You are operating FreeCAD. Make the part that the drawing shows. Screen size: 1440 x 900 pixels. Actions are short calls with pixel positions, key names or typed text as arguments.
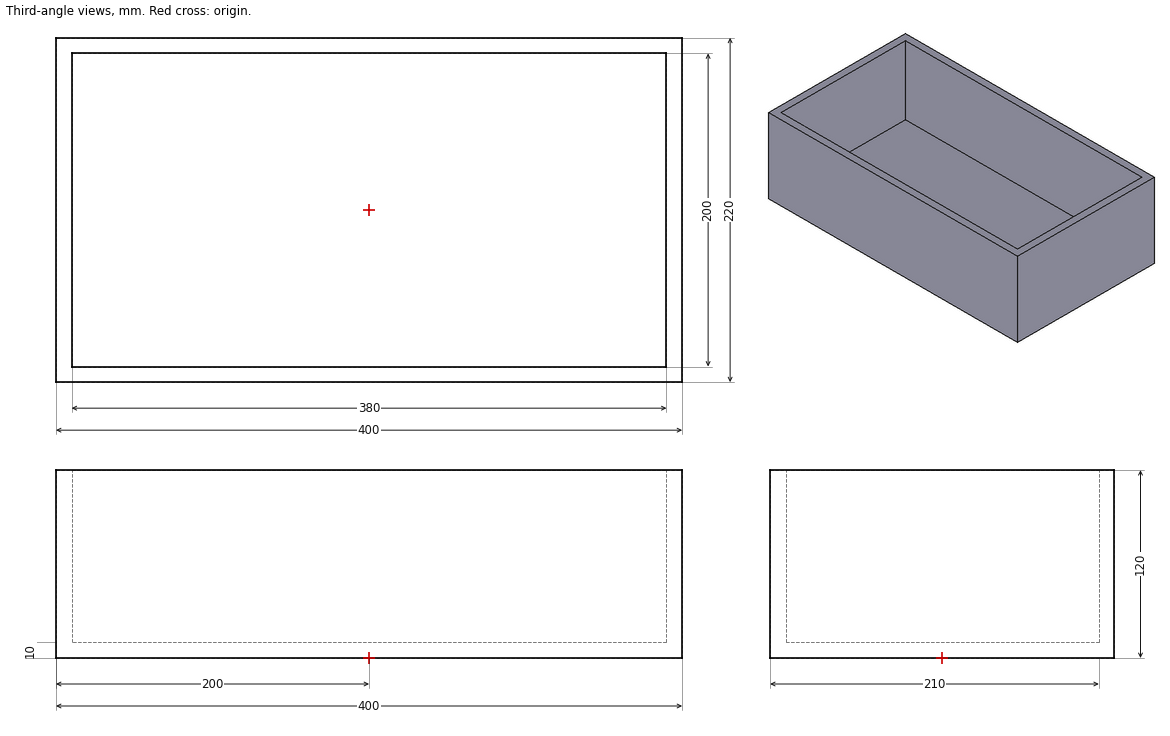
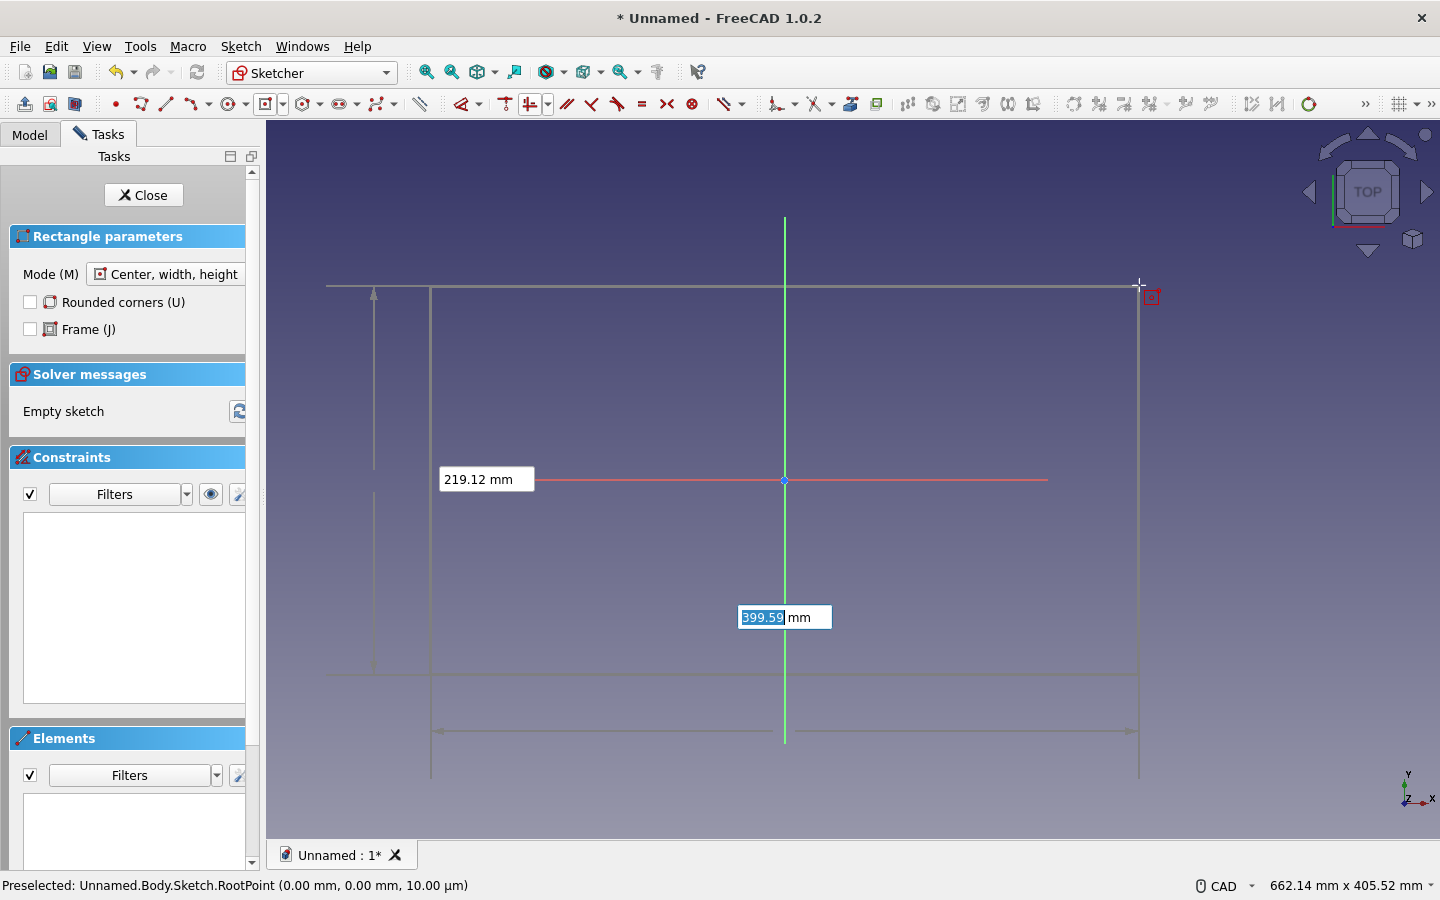
text(400)
key(Tab)
text(220)
key(Return)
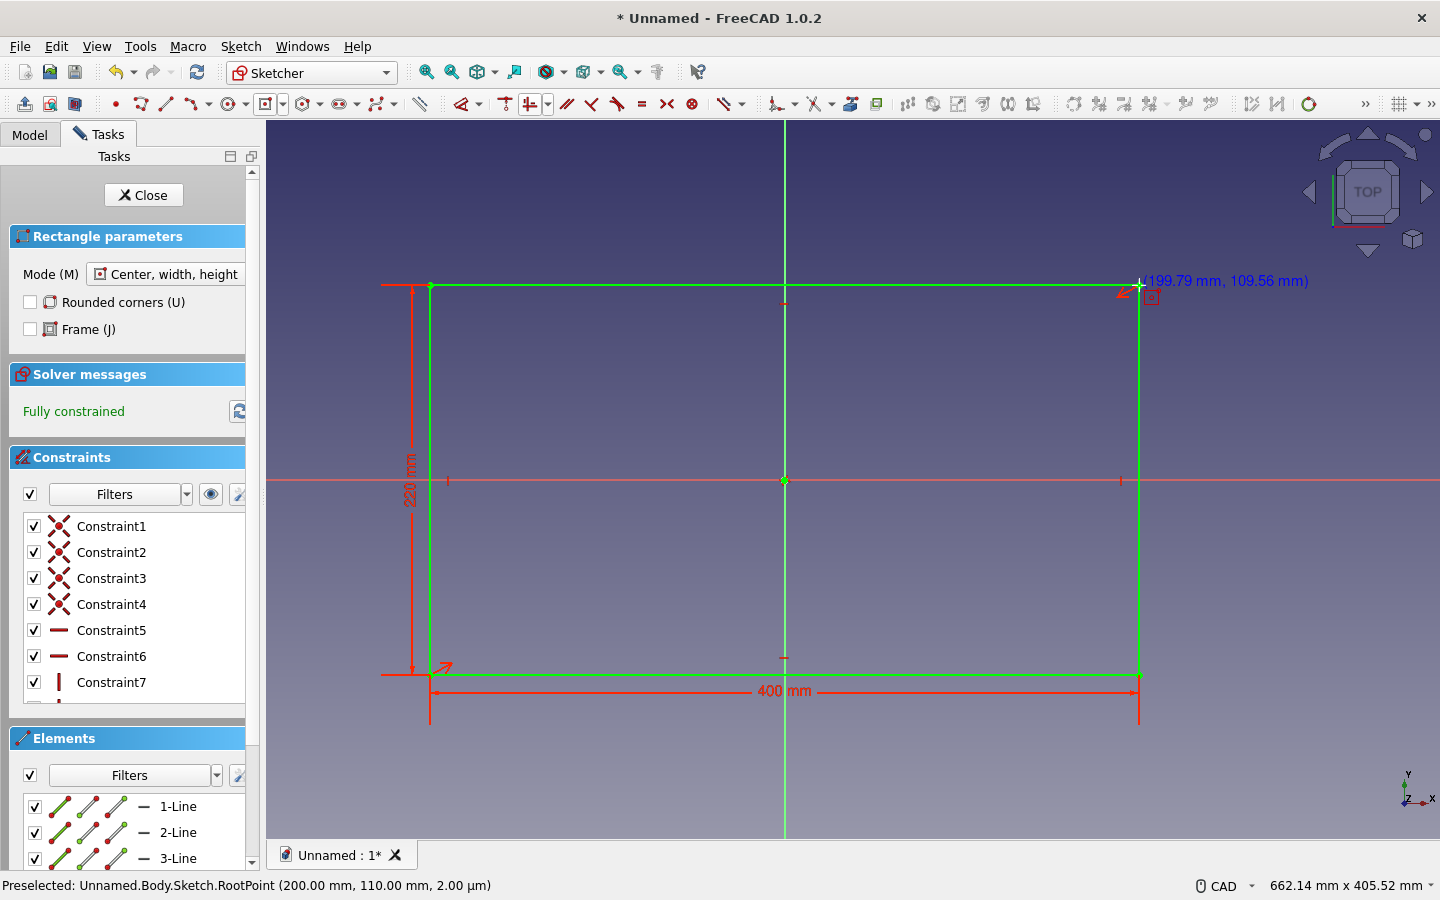
click(785, 480)
move(1122, 303)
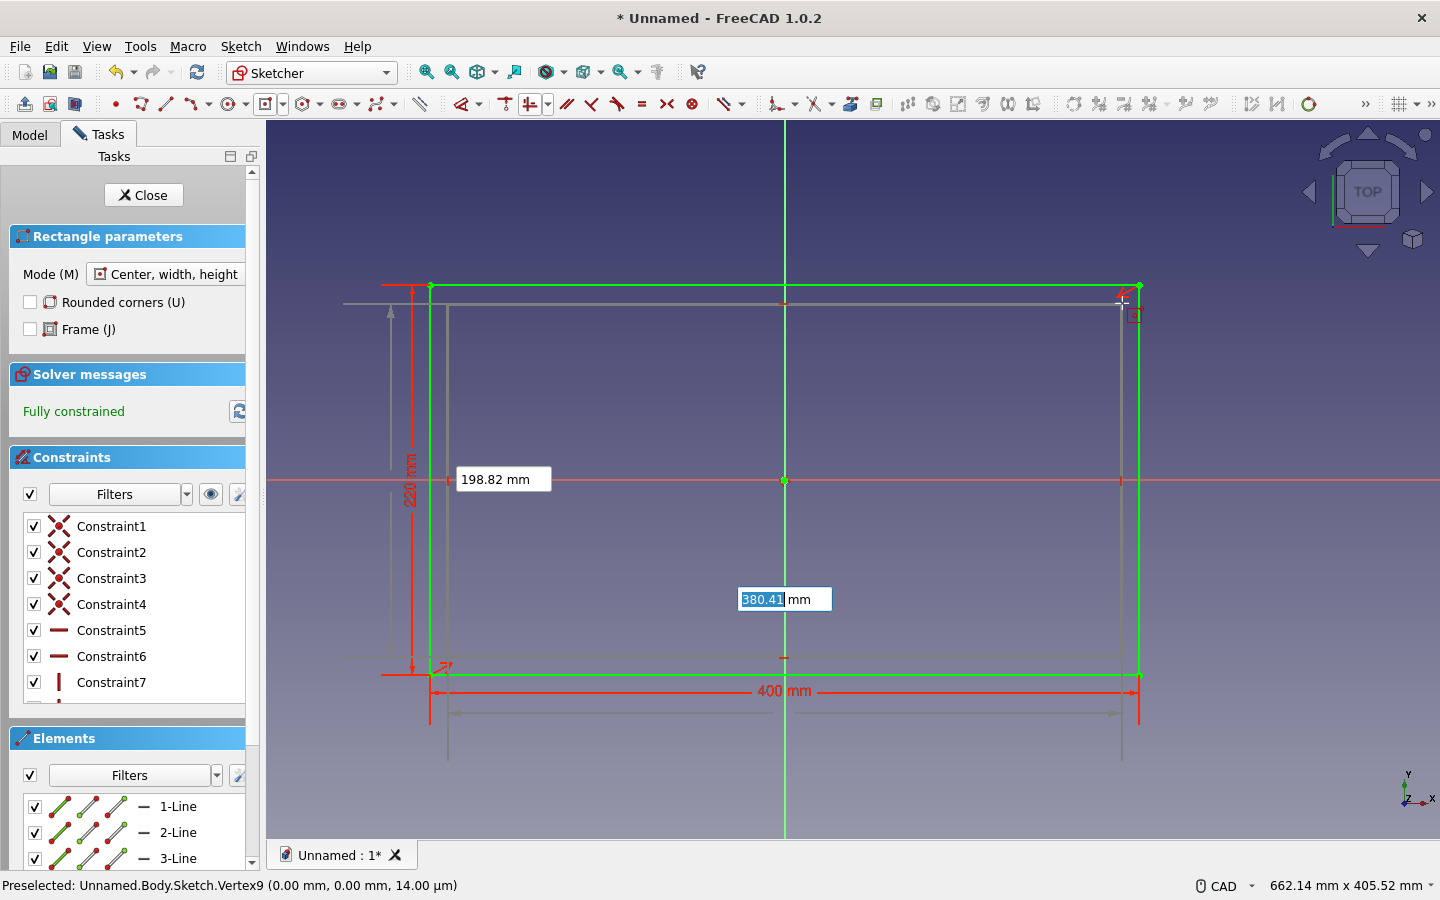
text(380)
key(Tab)
text(200)
key(Return)
key(Escape)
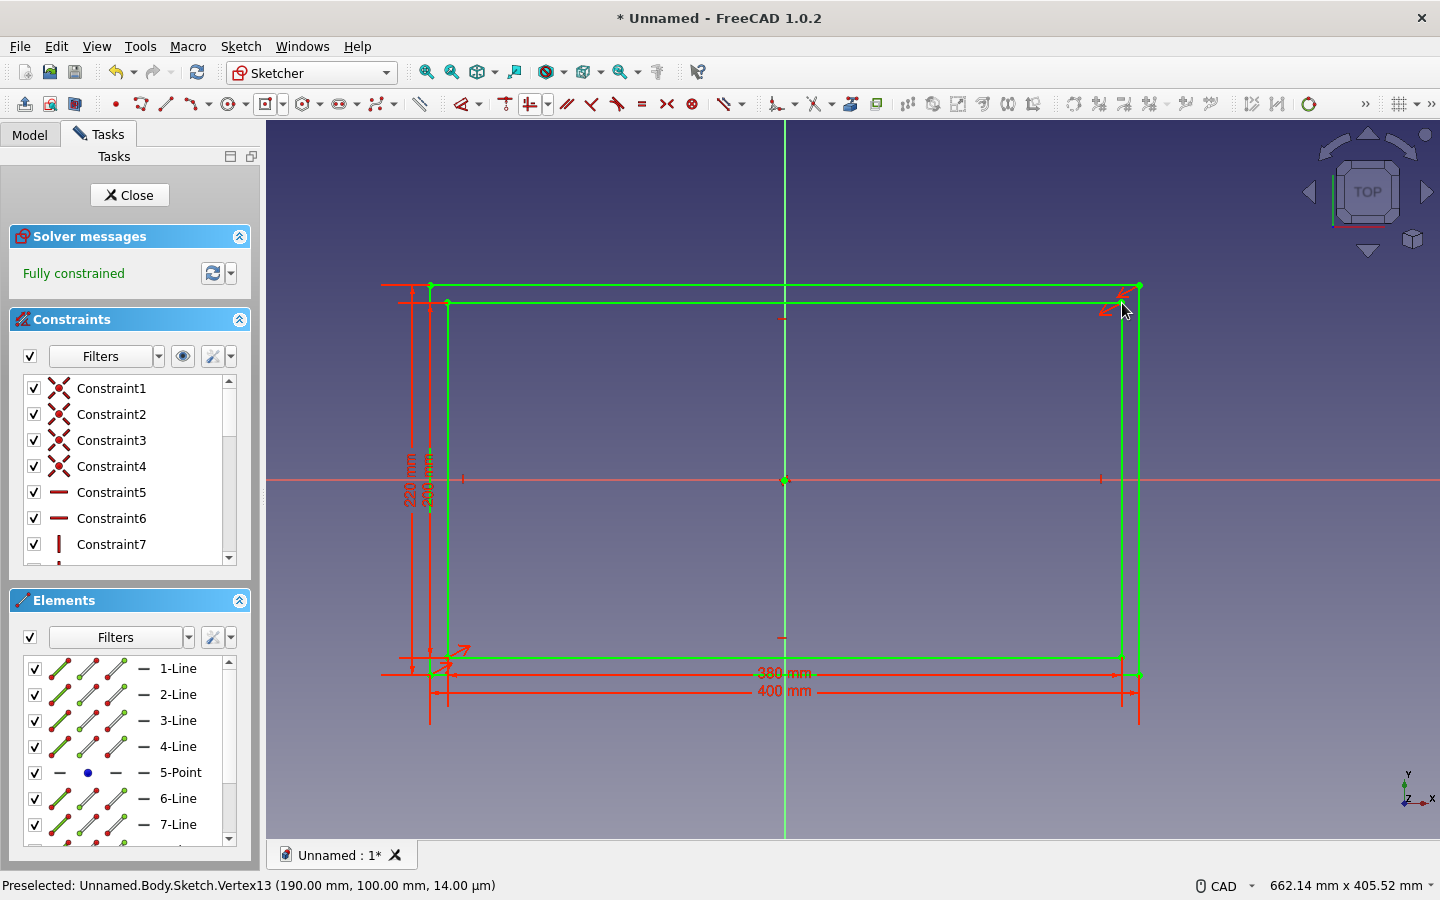
click(130, 195)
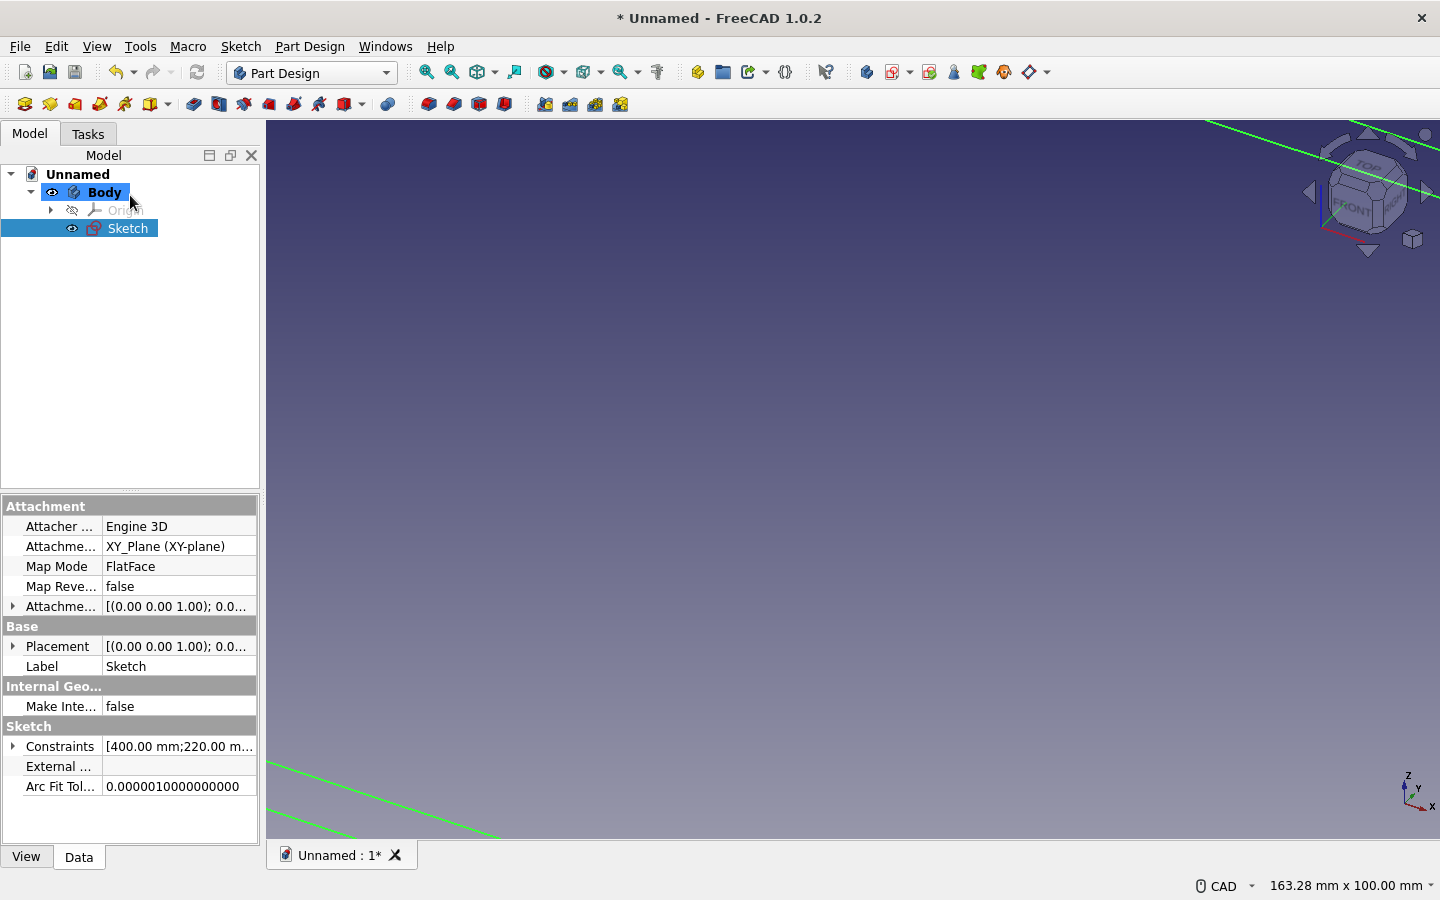
click(25, 104)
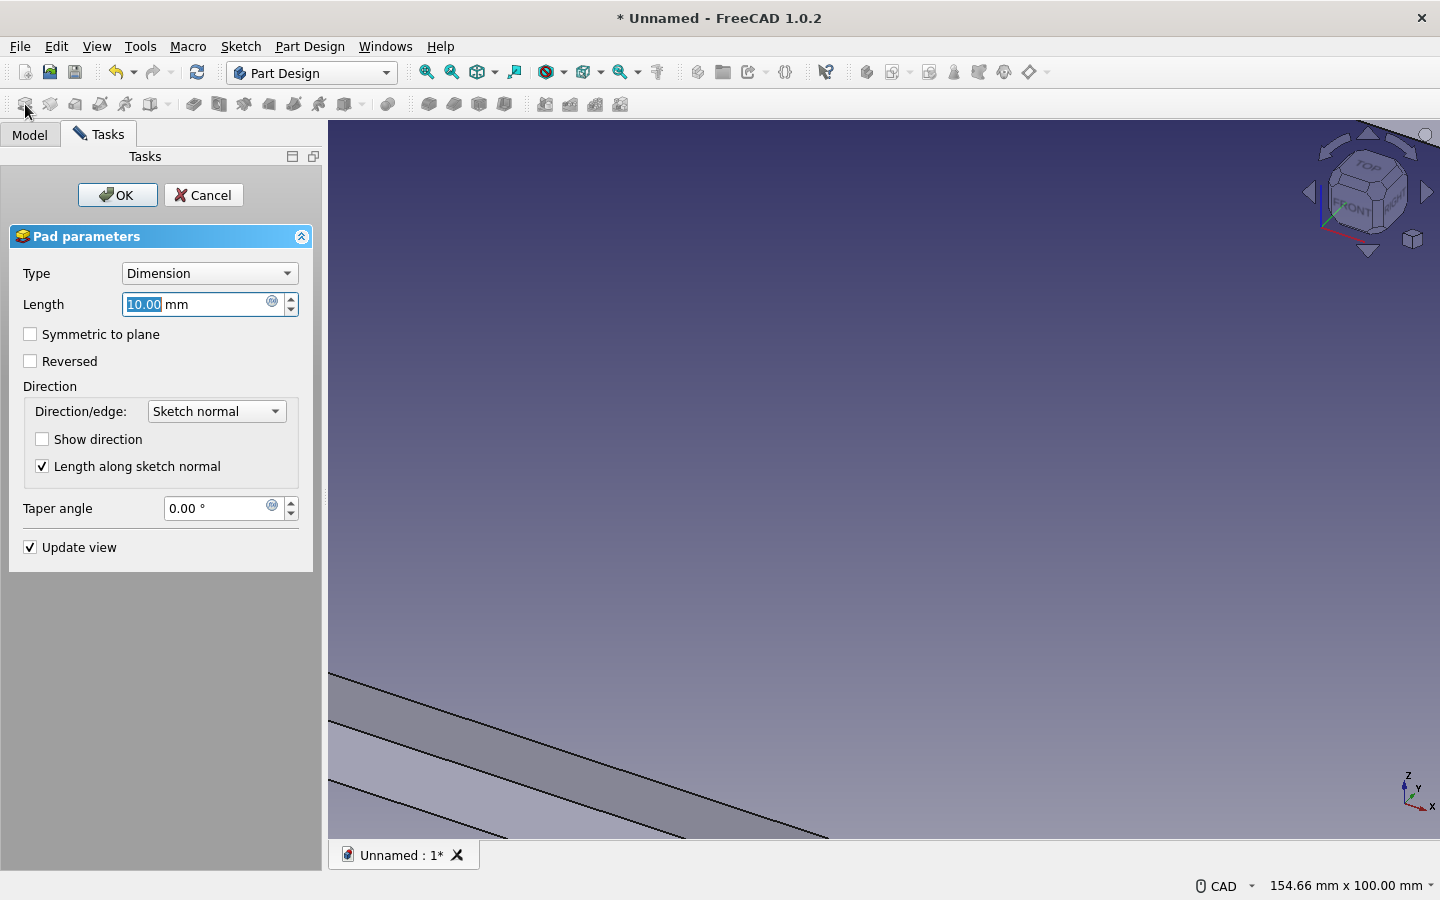
text(120)
key(Tab)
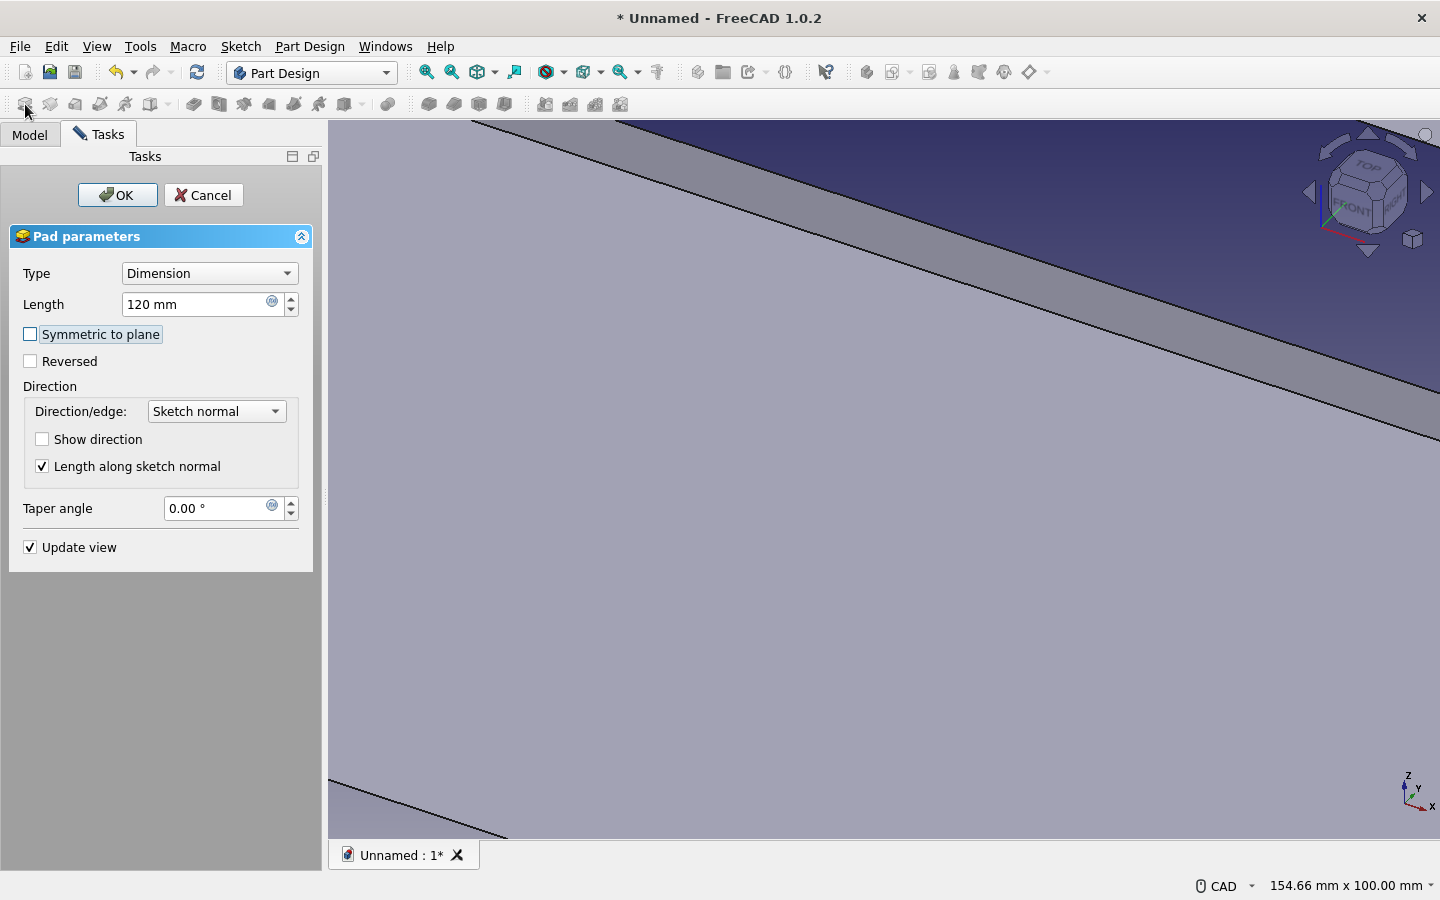
click(118, 195)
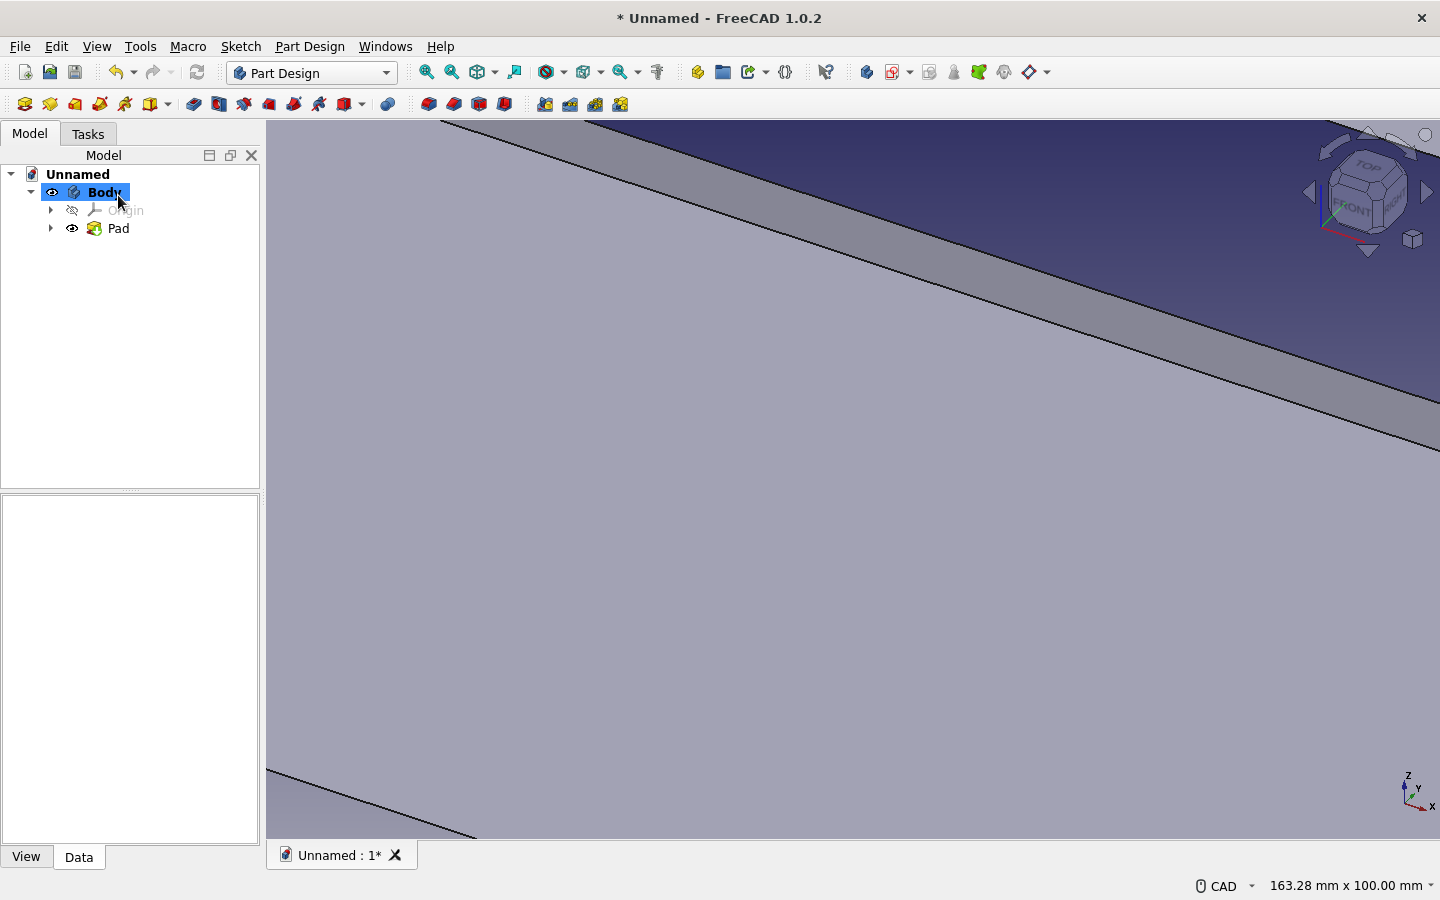
click(427, 72)